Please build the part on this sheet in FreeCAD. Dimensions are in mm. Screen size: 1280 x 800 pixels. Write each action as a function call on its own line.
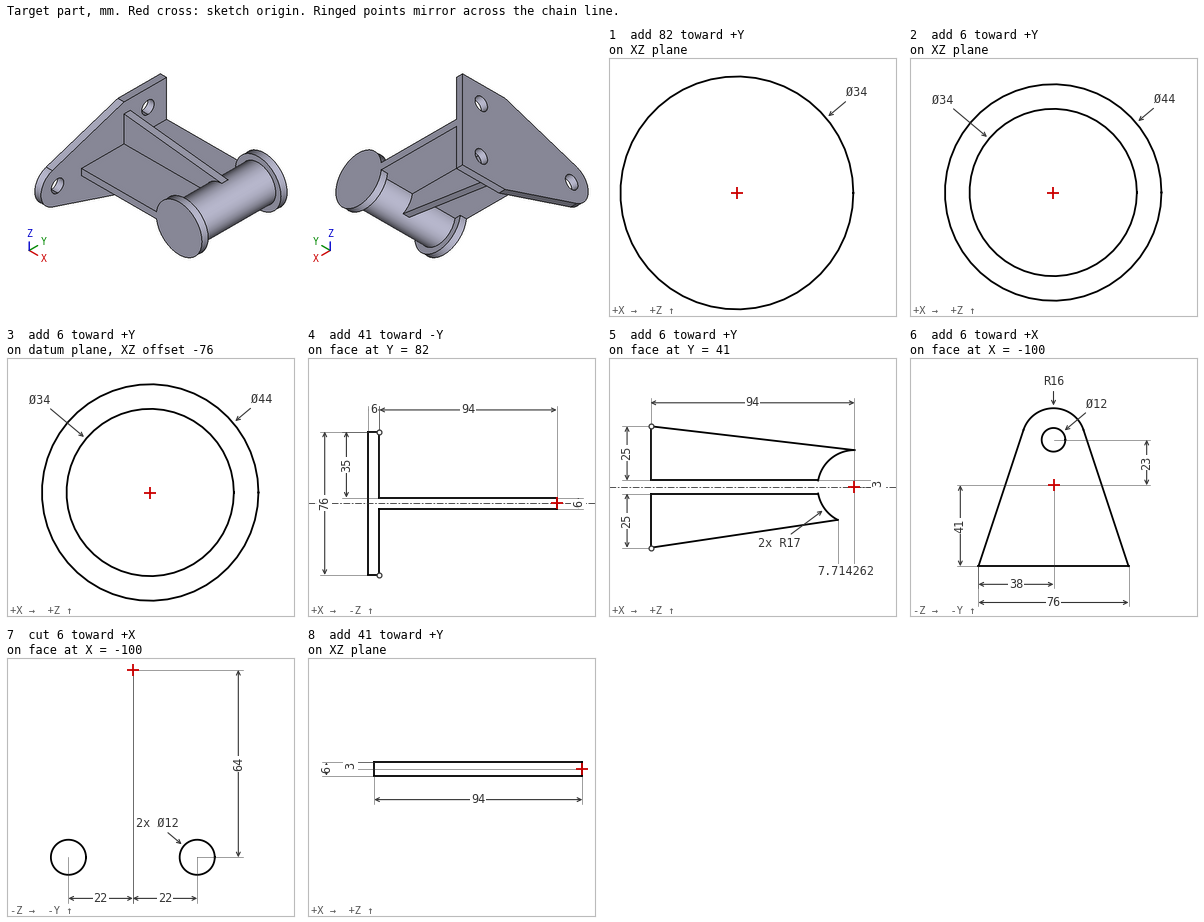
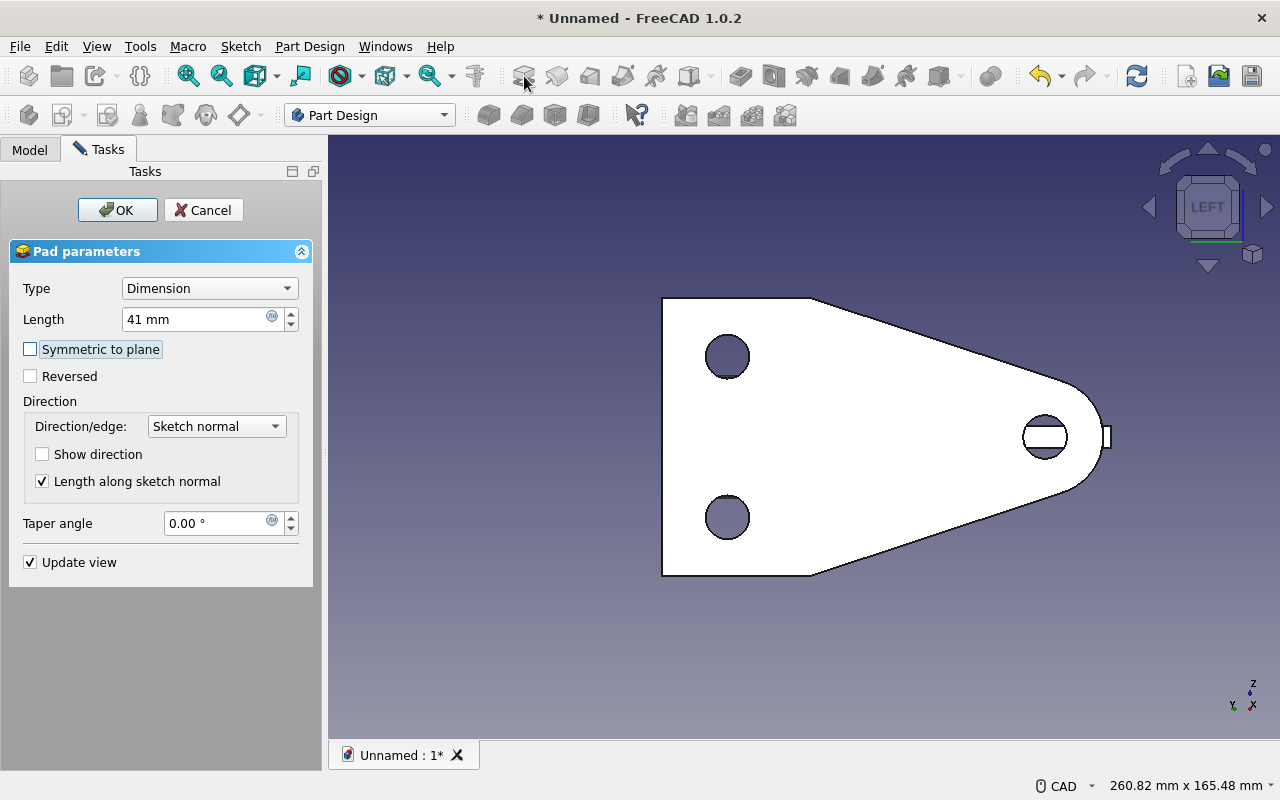
click(31, 376)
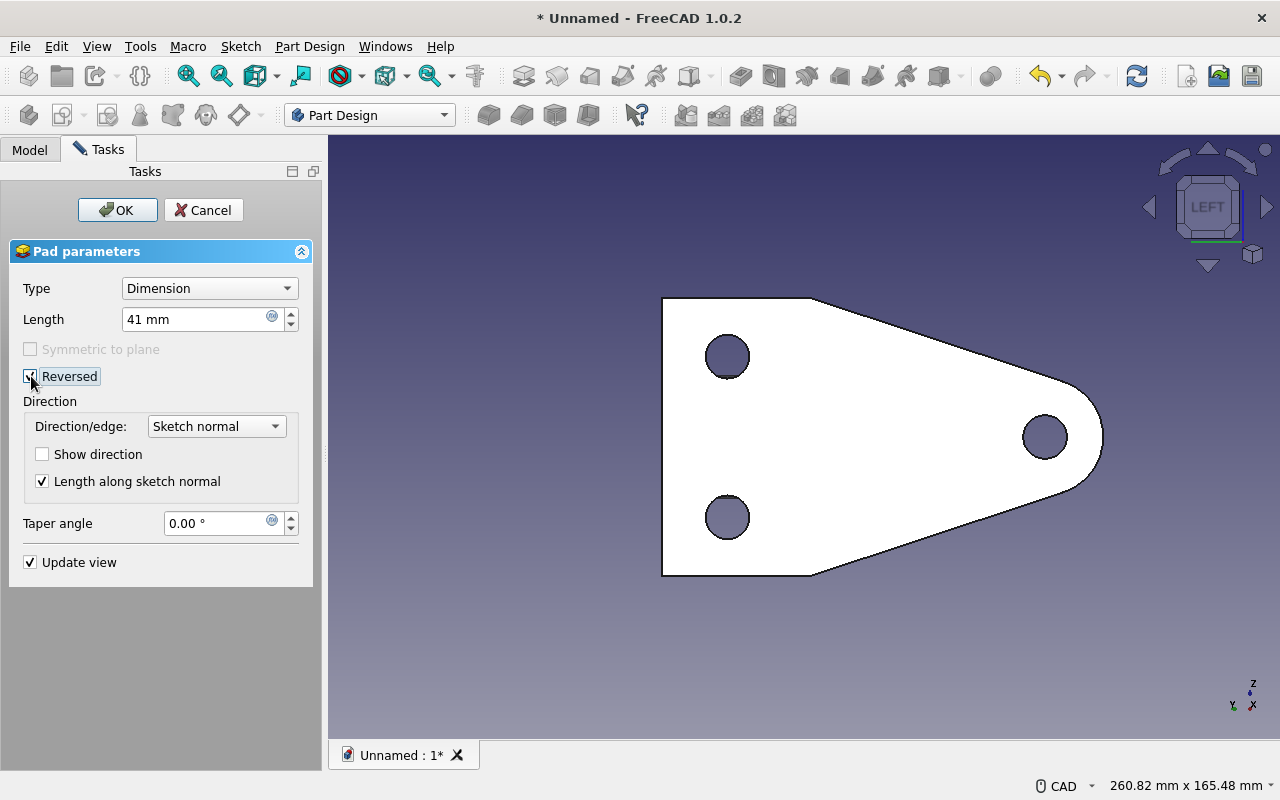
click(118, 210)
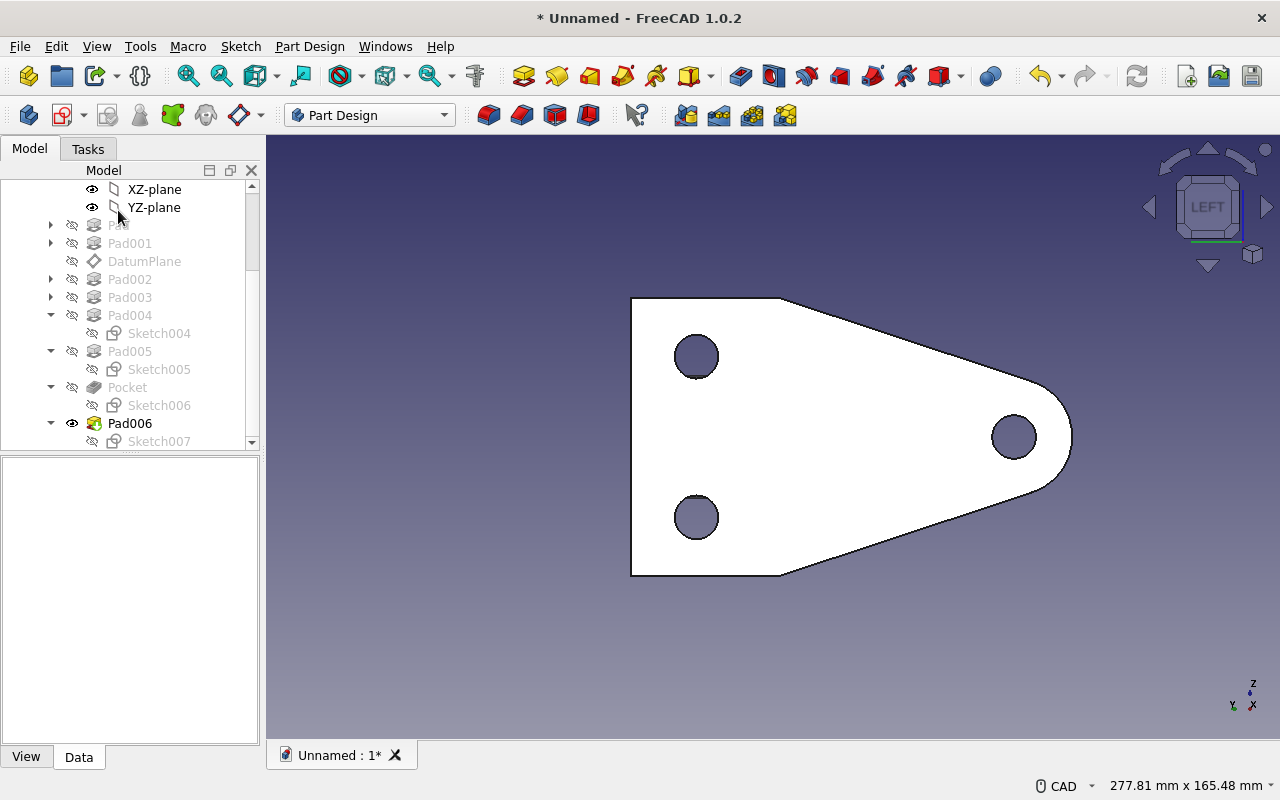
key(0)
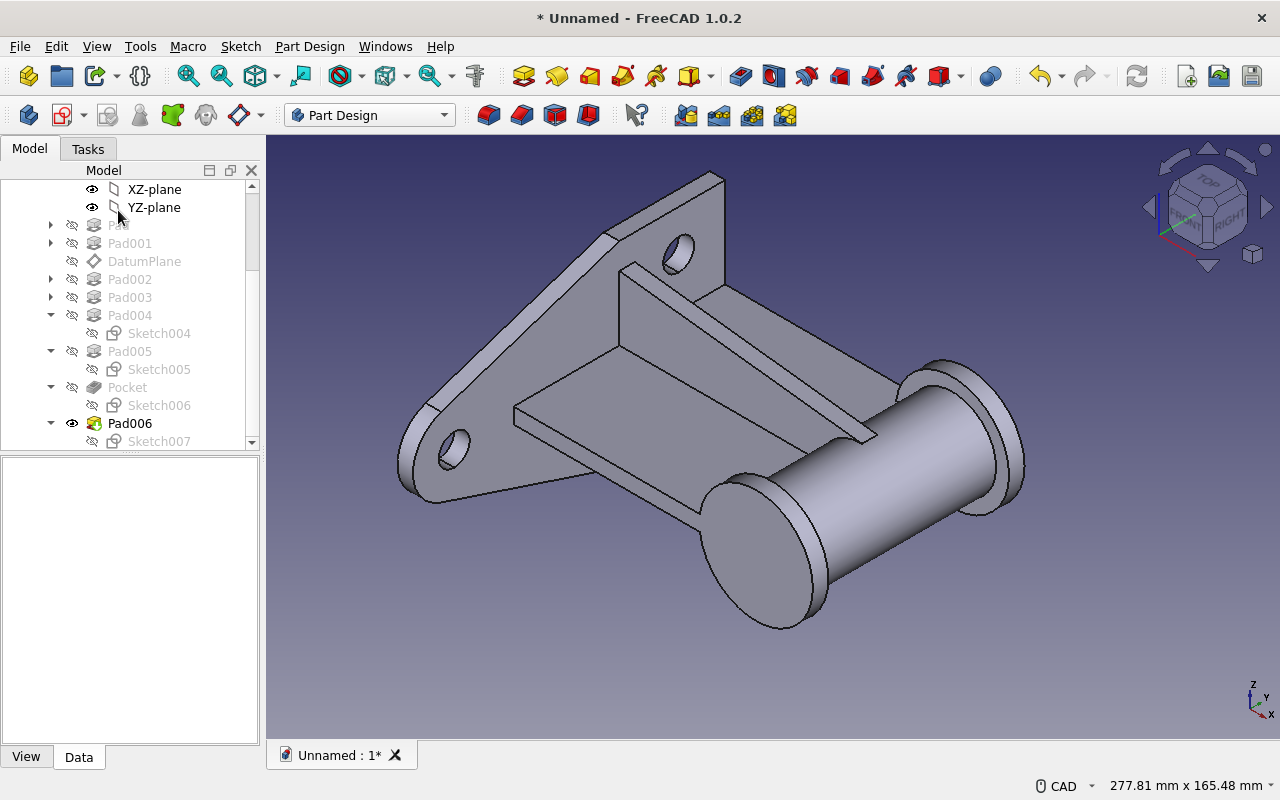
click(189, 76)